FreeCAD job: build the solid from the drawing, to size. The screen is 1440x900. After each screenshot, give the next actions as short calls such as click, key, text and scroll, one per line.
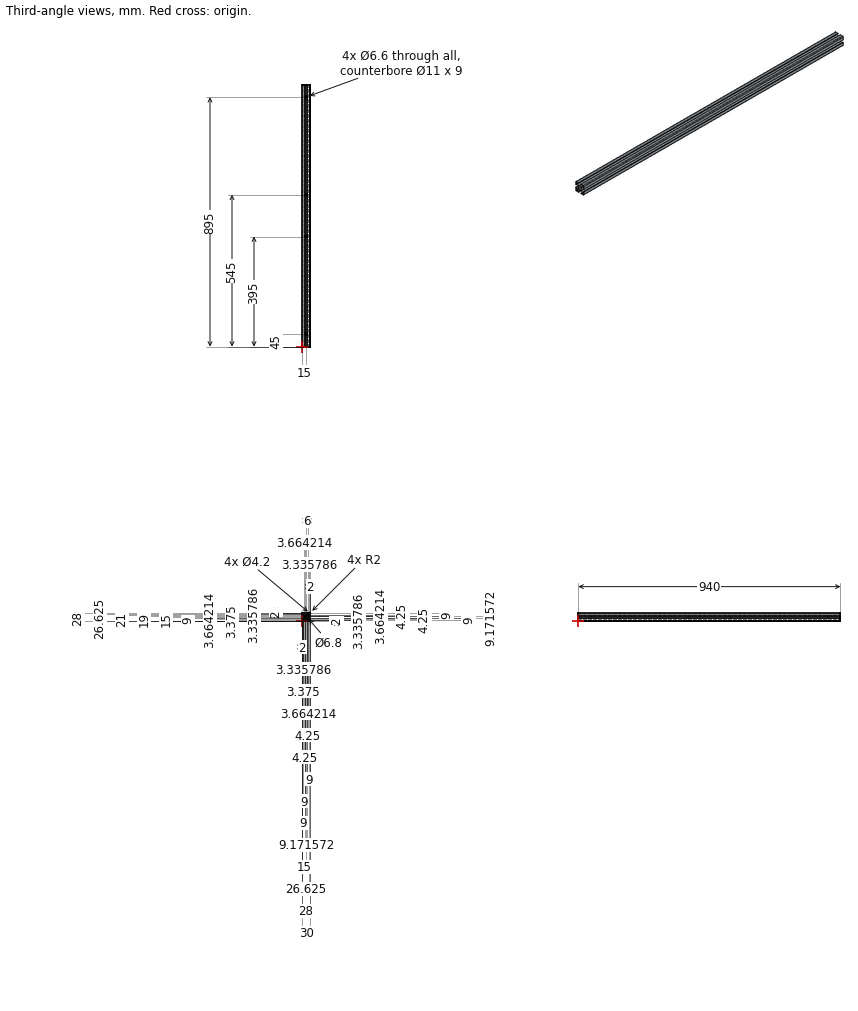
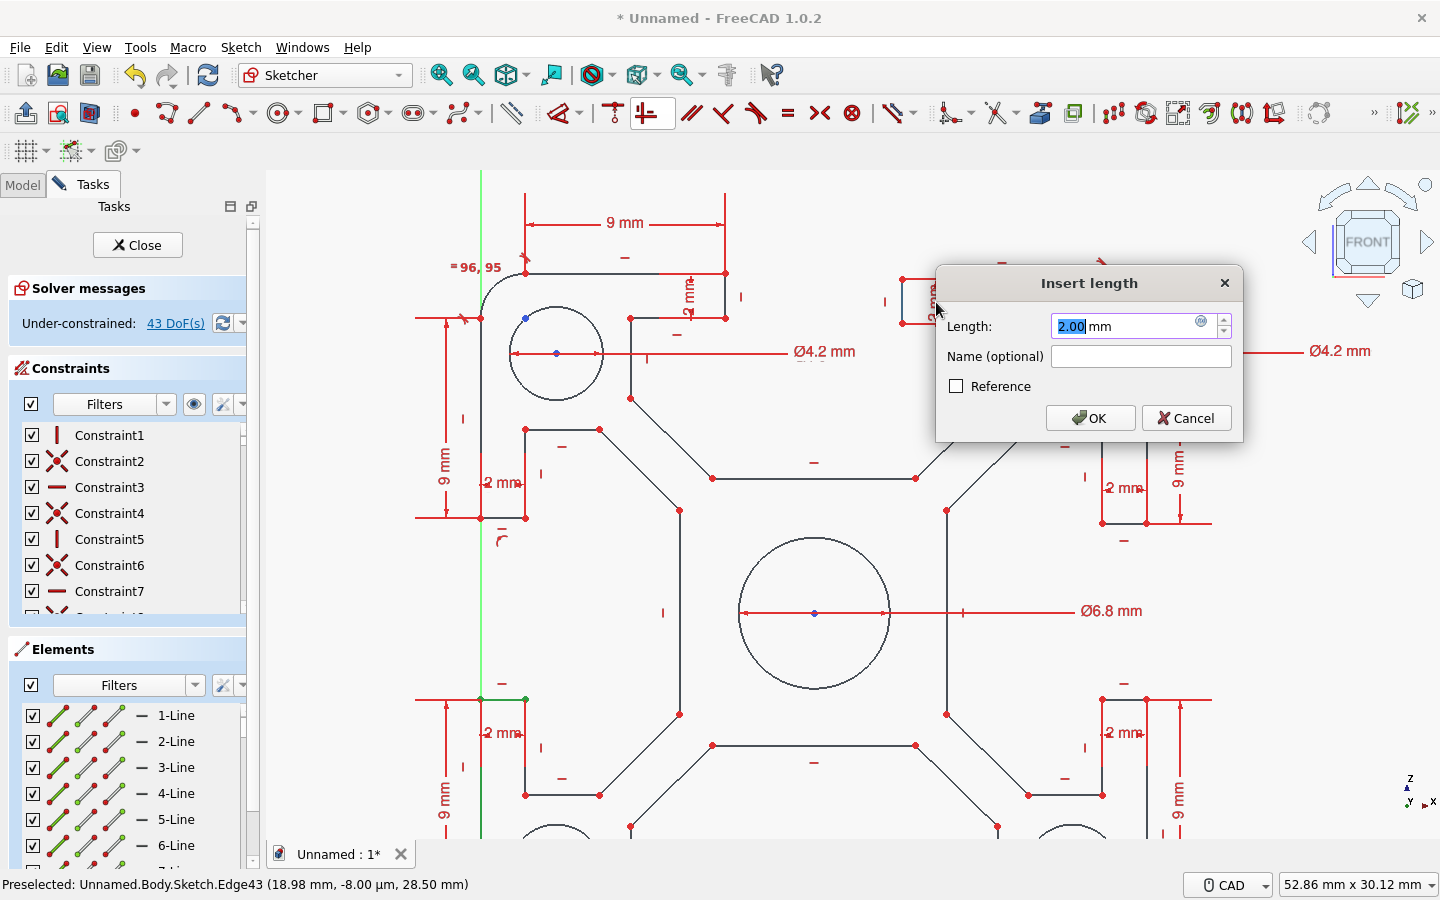
text(2)
key(Return)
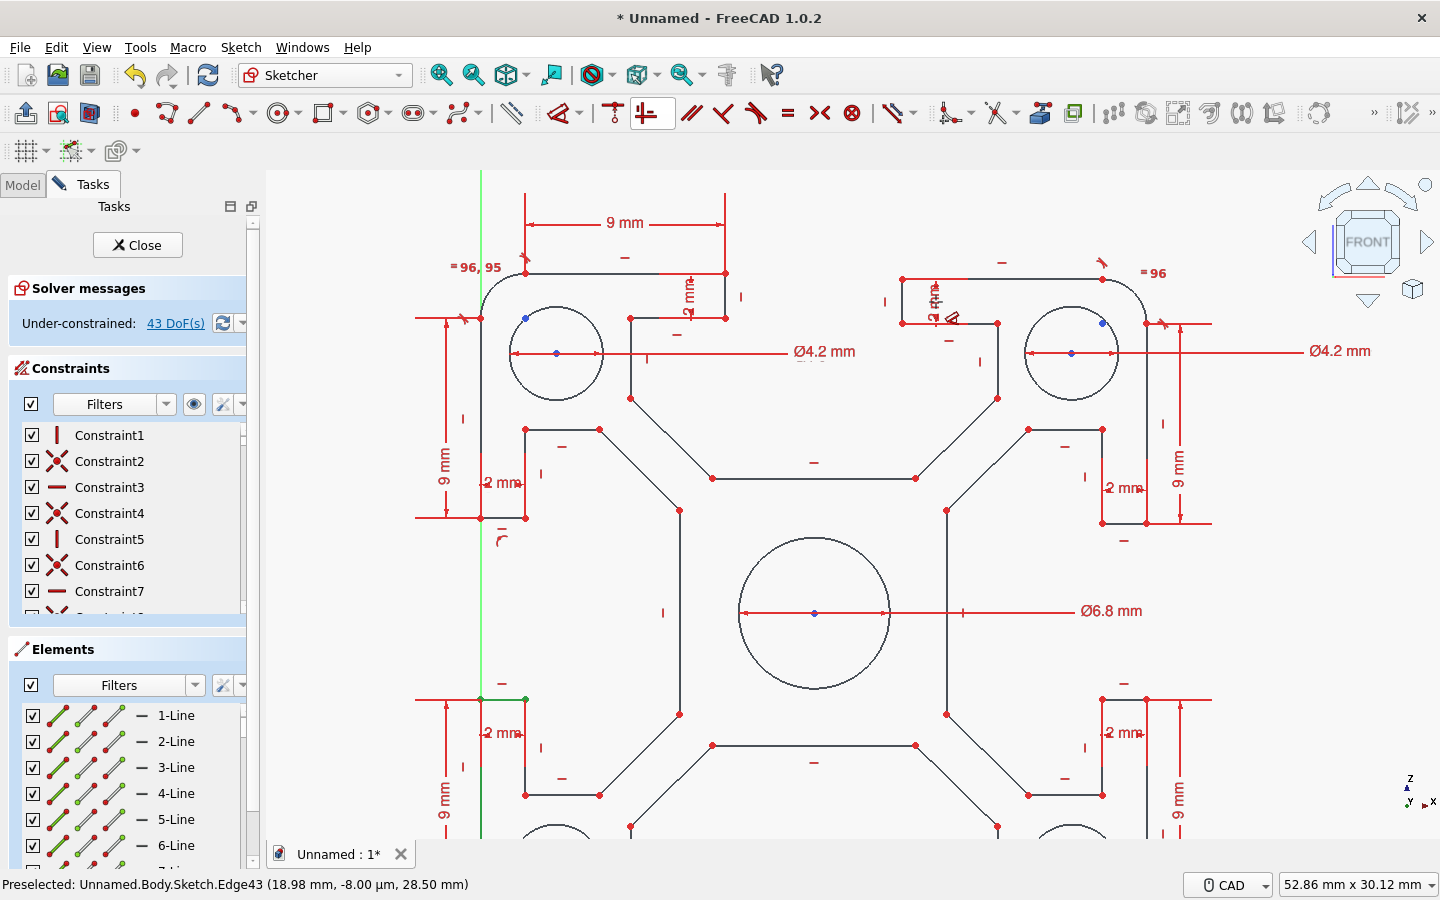
click(962, 279)
click(1002, 245)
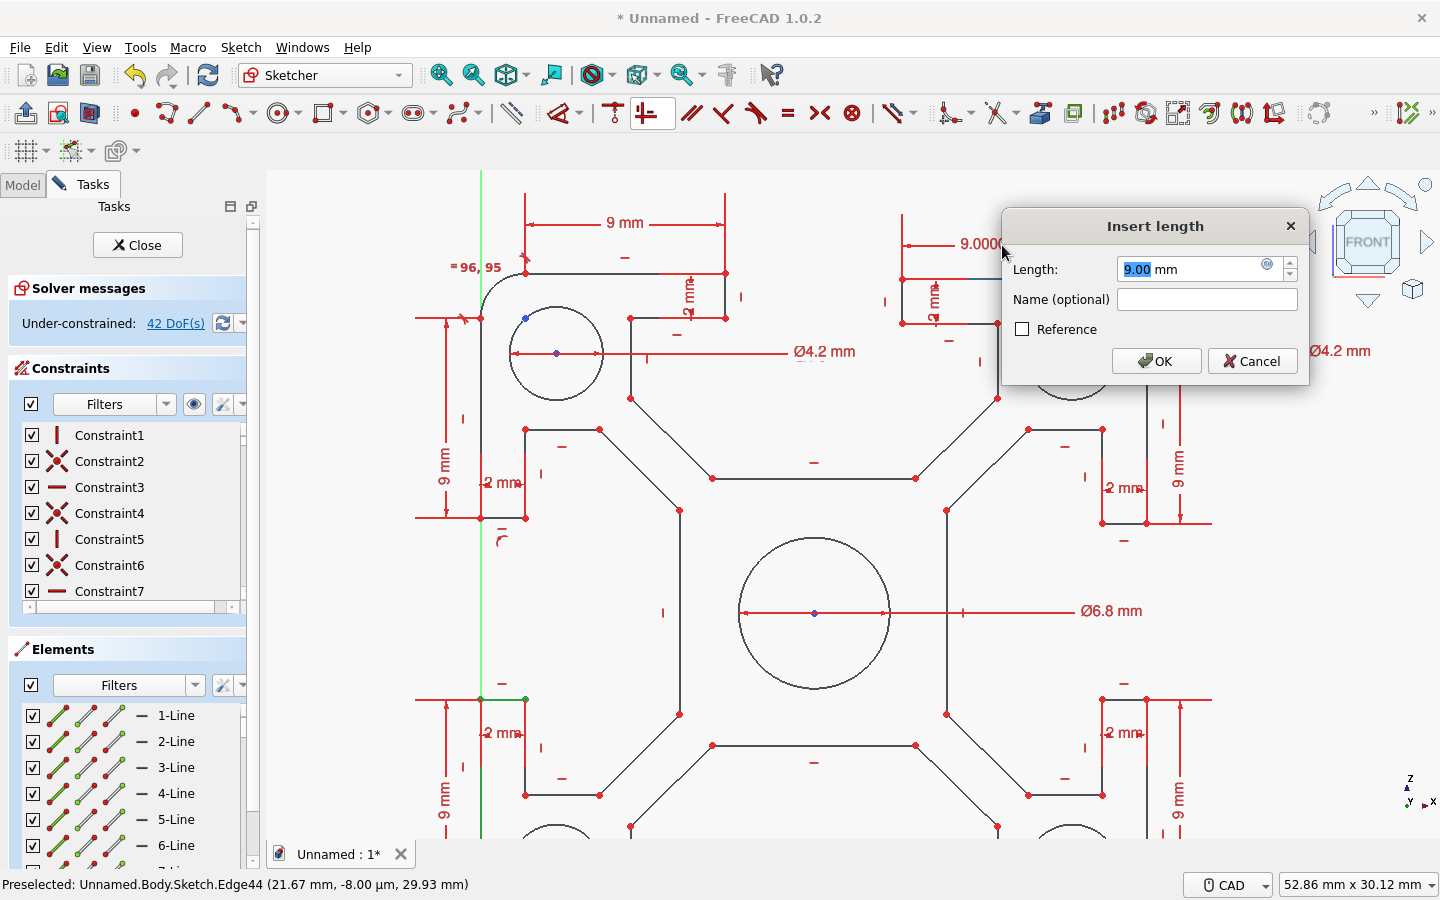
text(9)
key(Return)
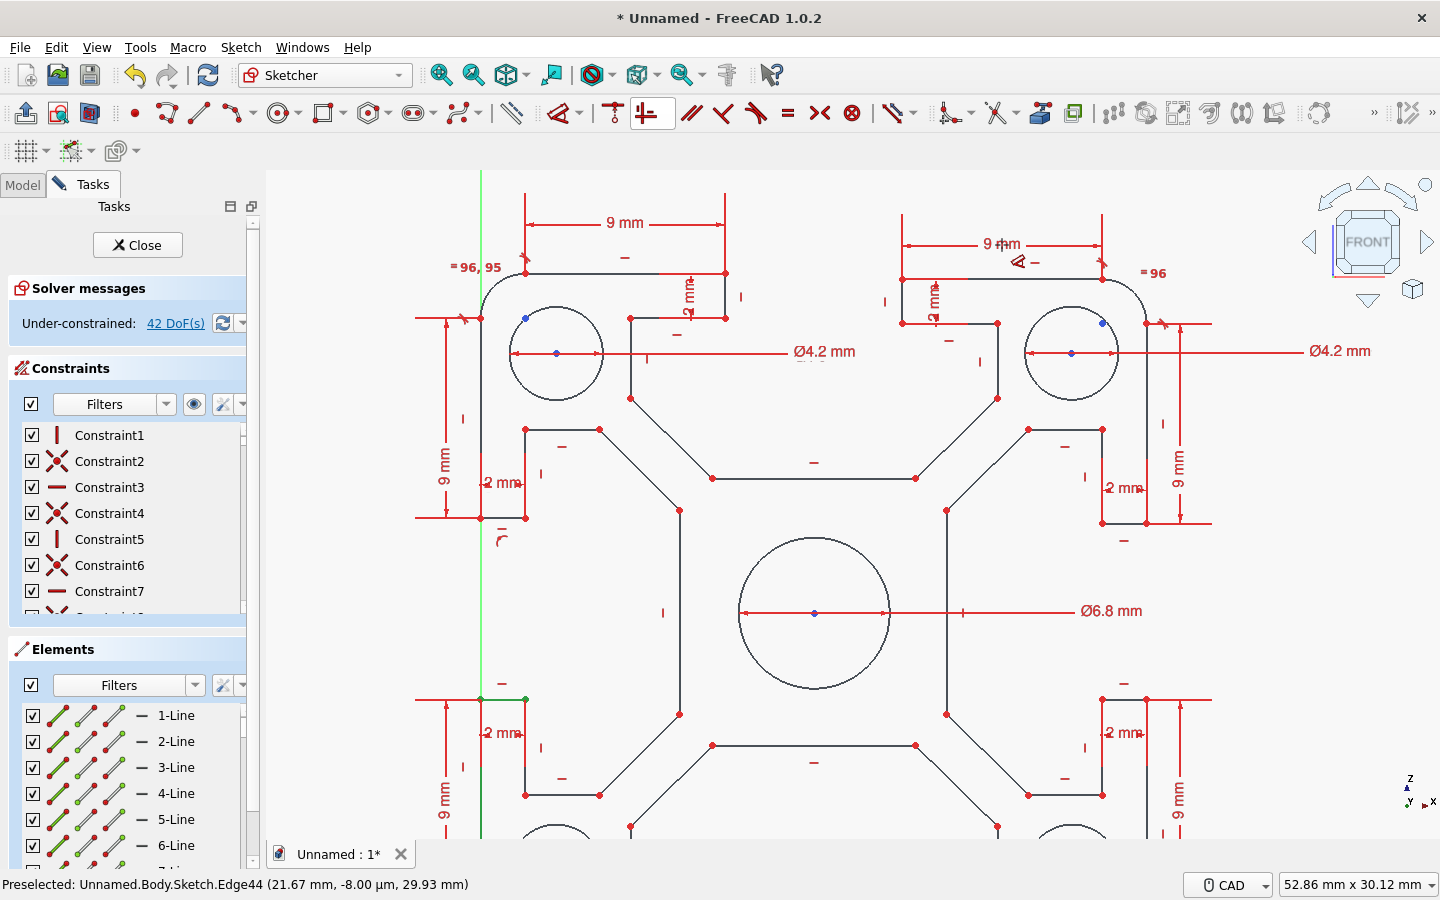
click(916, 746)
click(447, 778)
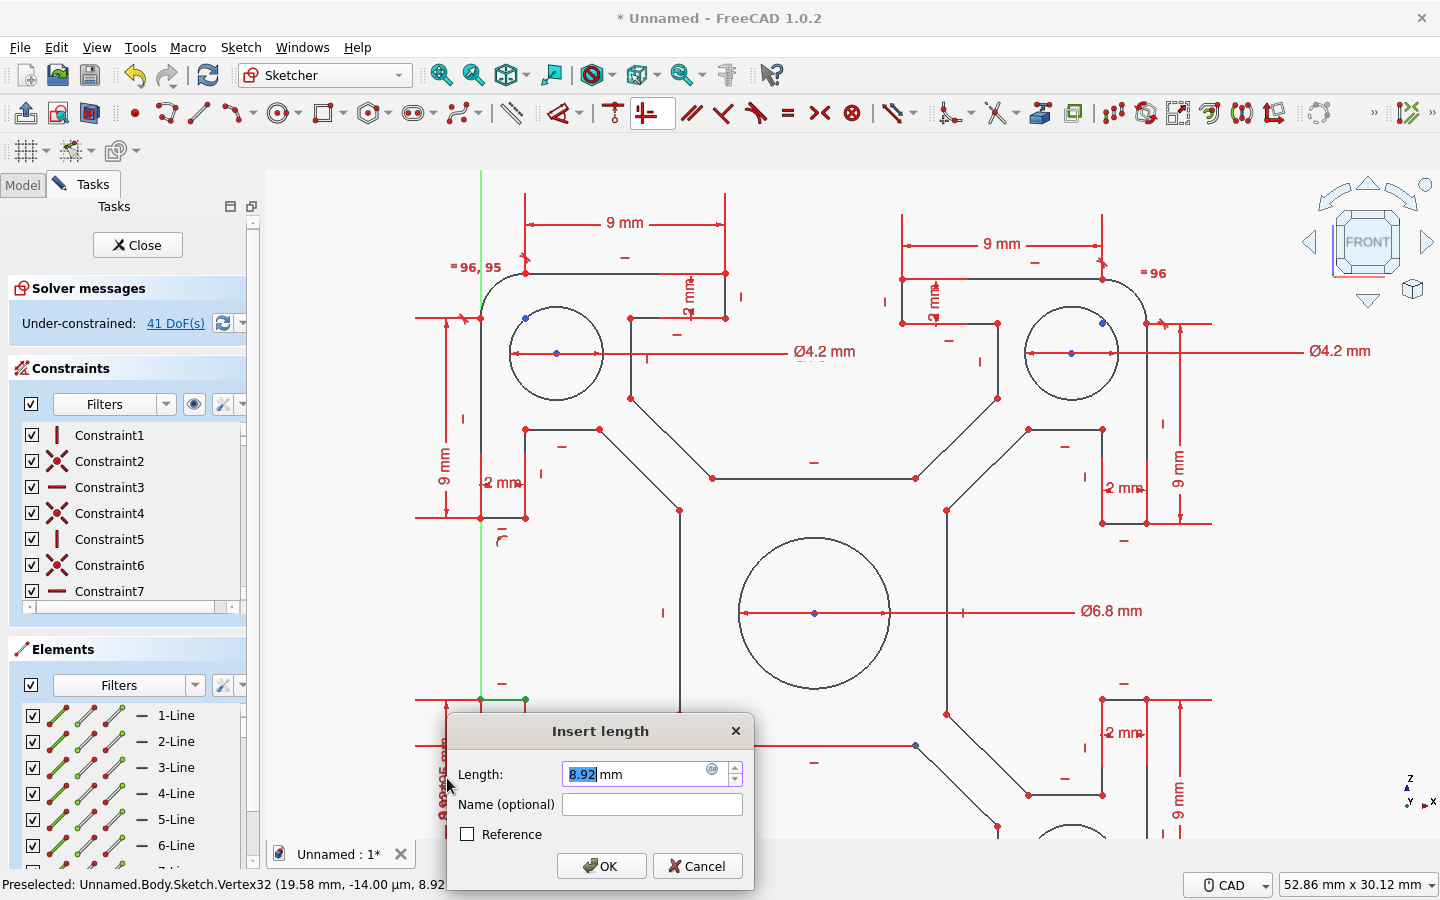
text(9)
key(Return)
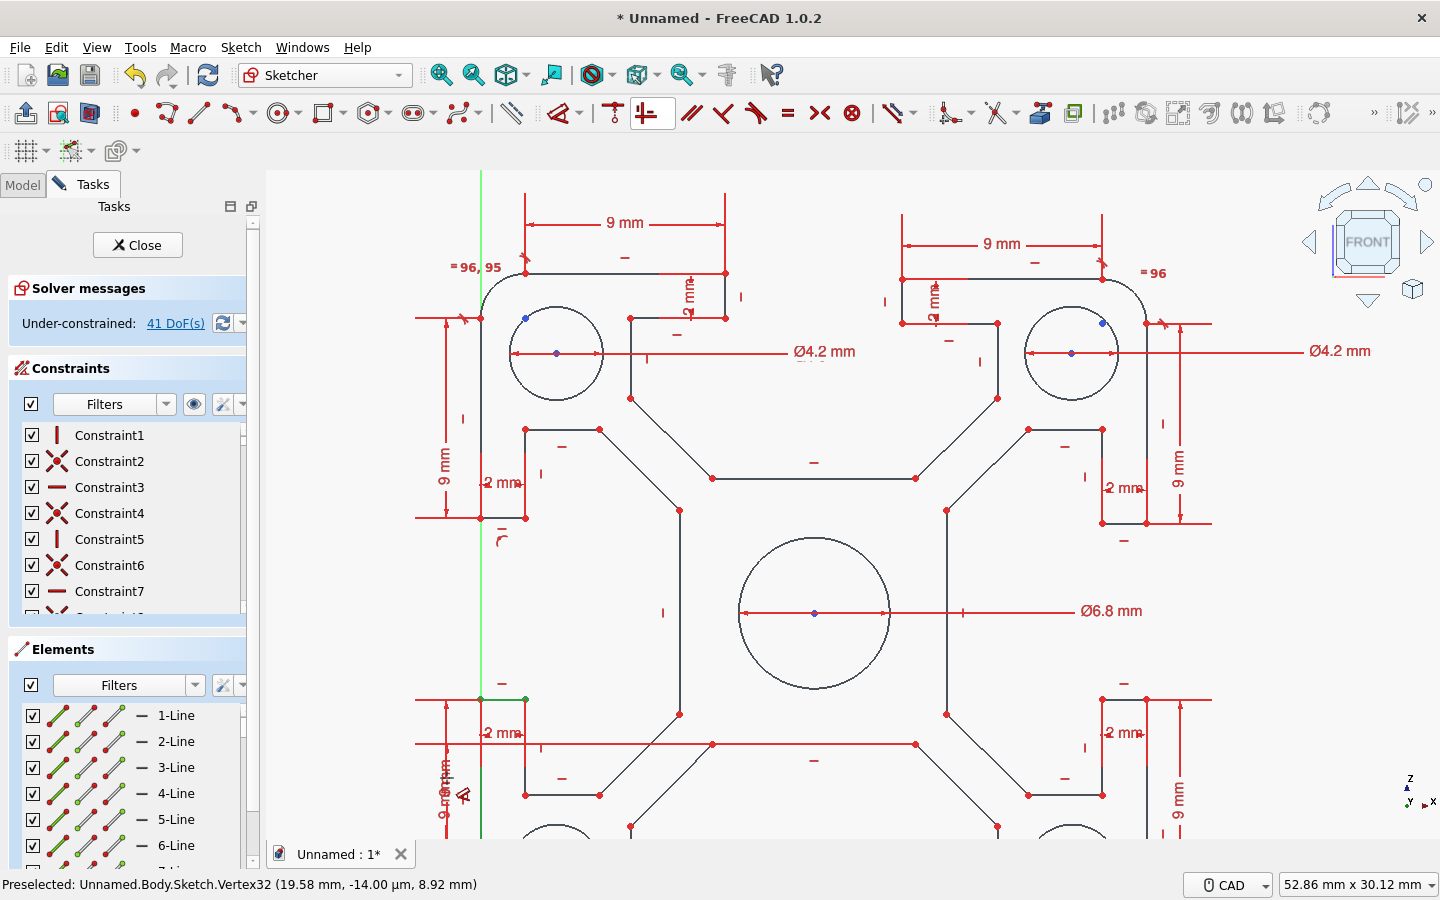
click(680, 715)
click(580, 681)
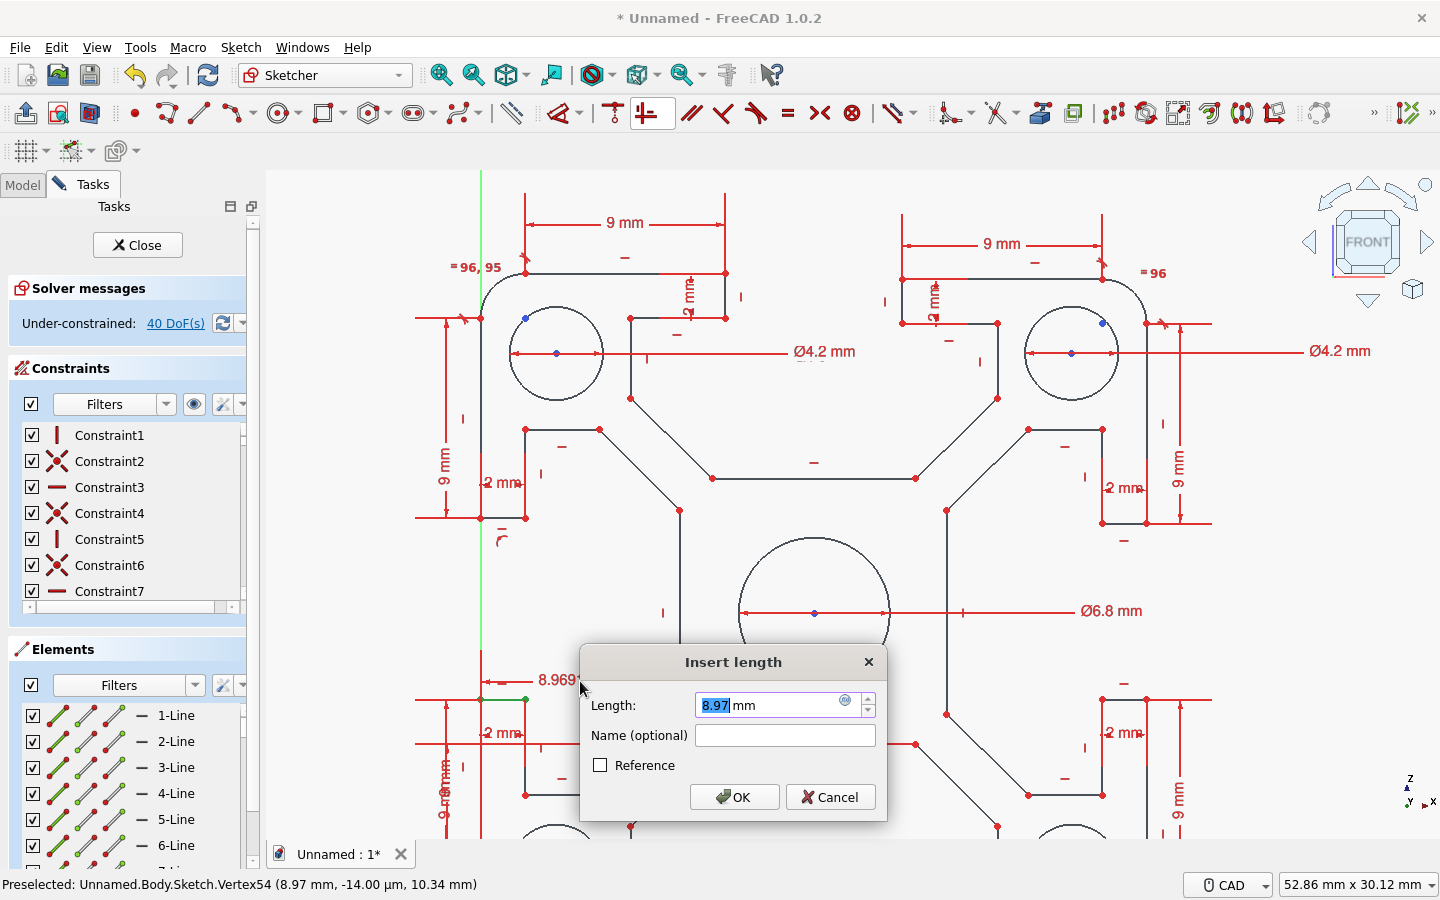
text(9)
key(Return)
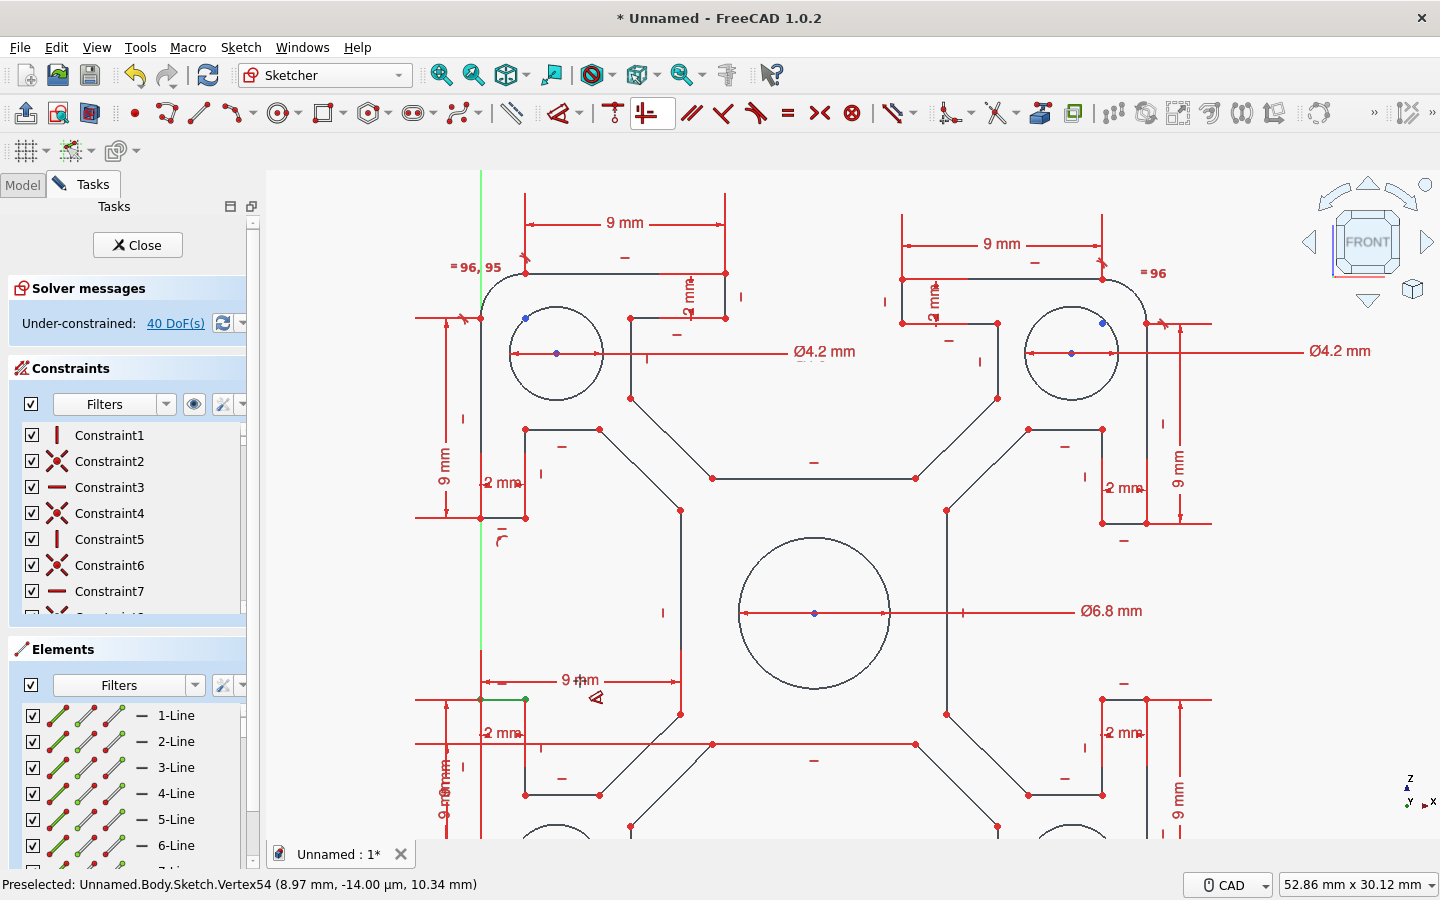
click(814, 613)
click(648, 579)